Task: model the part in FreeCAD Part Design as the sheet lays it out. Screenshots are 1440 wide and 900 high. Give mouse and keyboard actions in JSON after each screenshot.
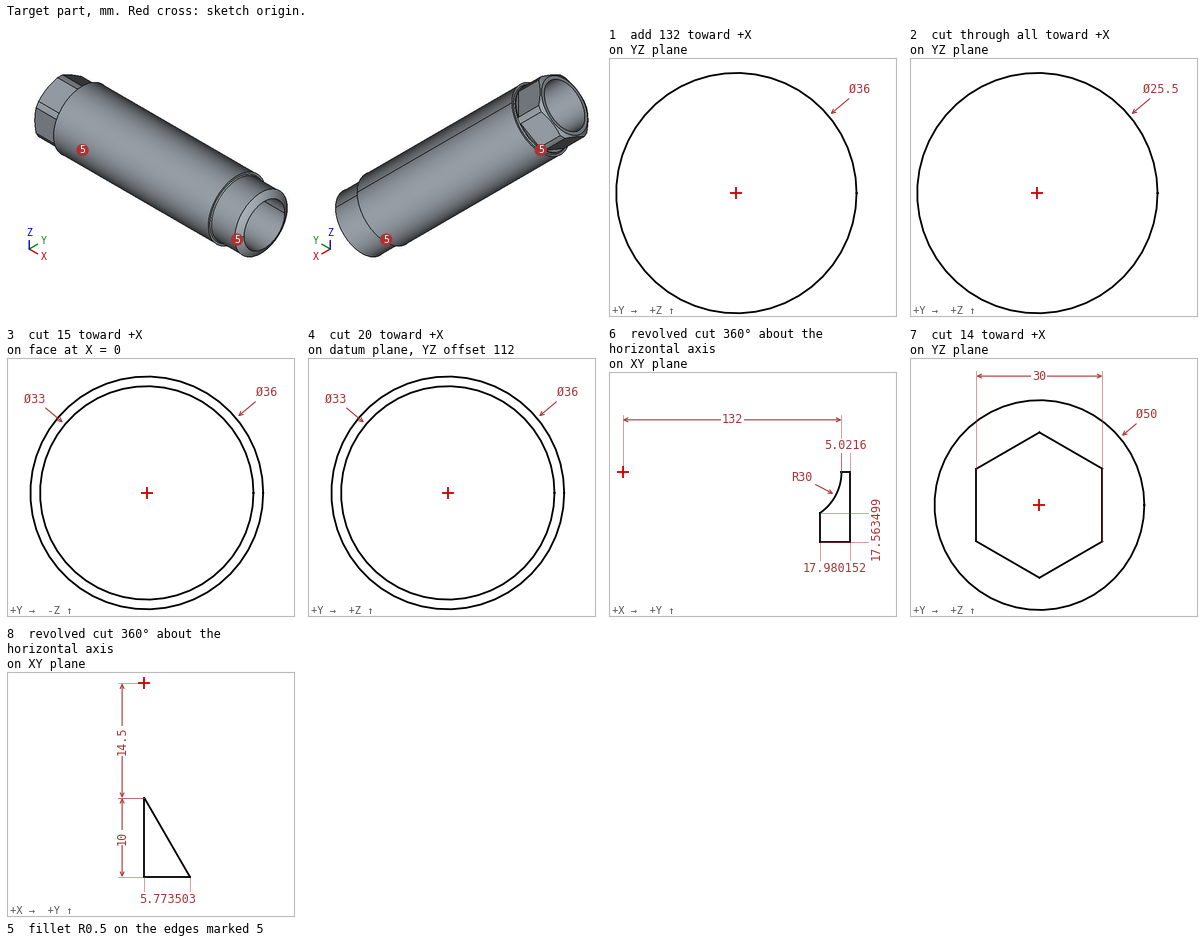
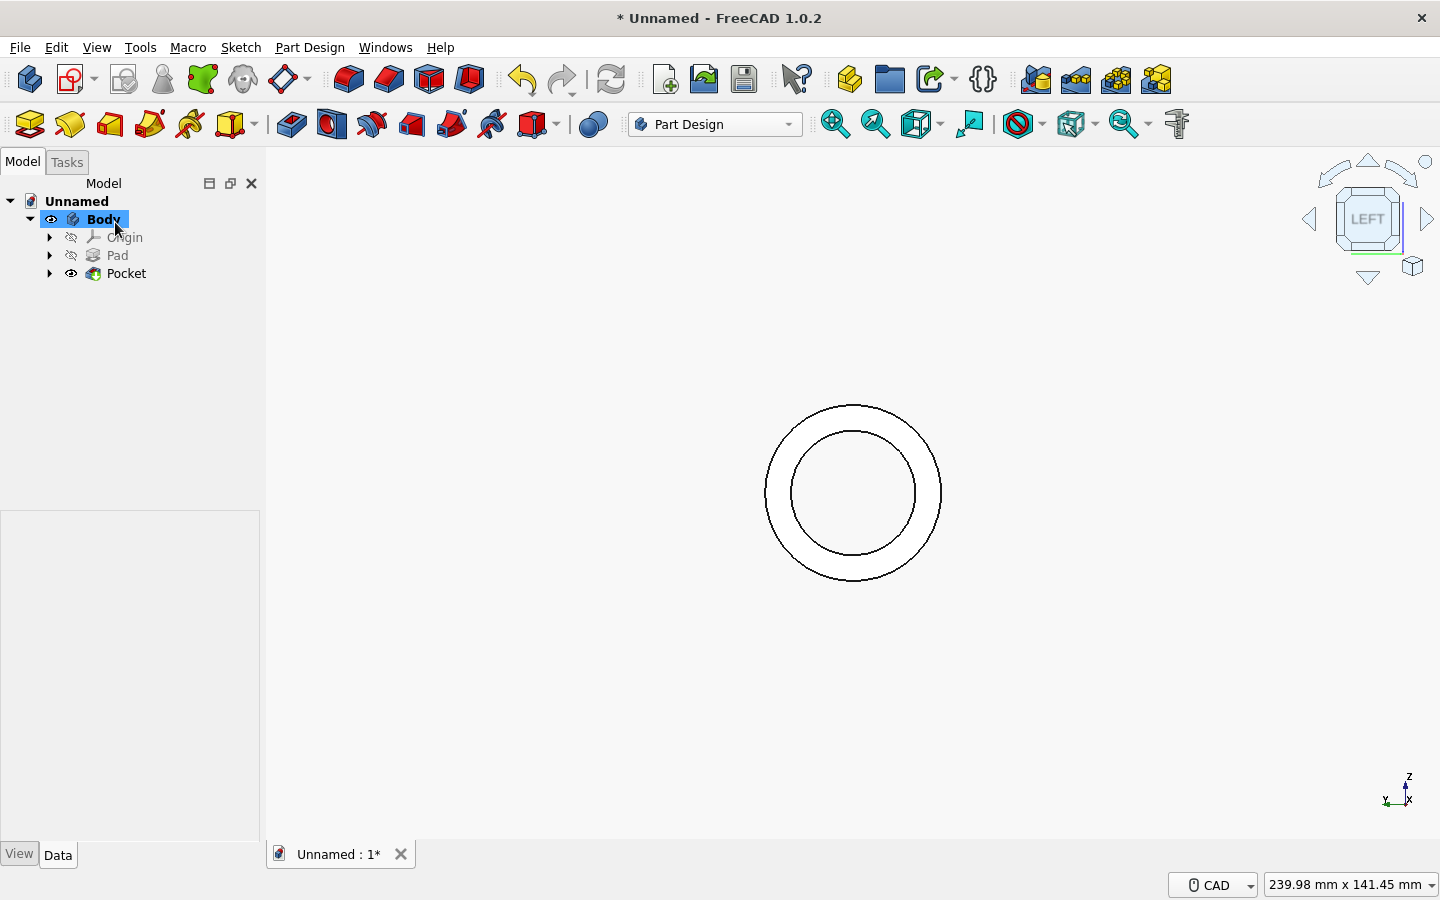
{"action": "key", "text": "v f"}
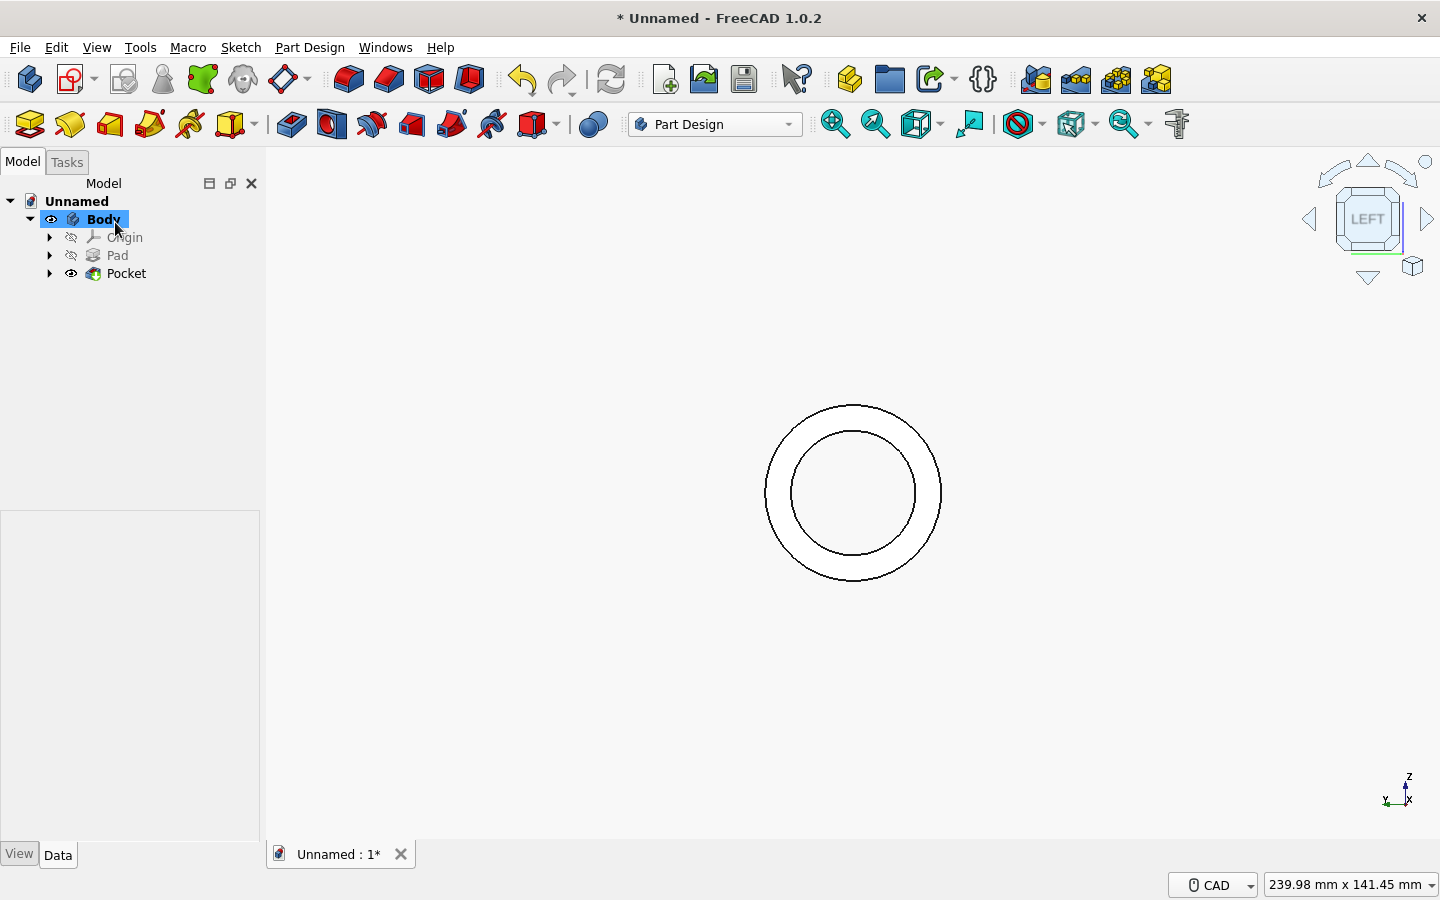
{"action": "left_click", "coordinate": [778, 492]}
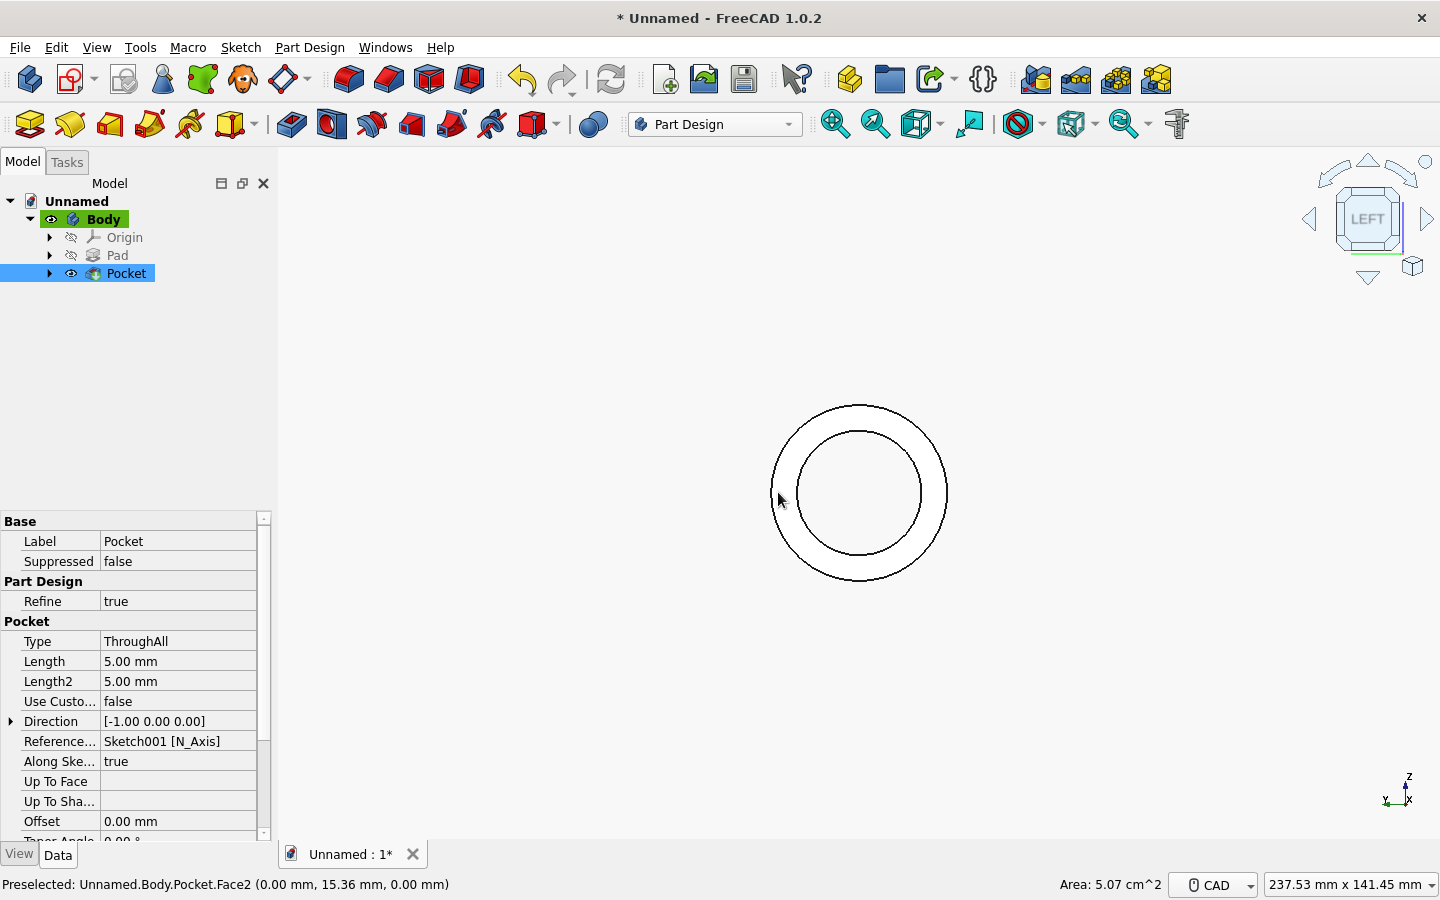
{"action": "left_click", "coordinate": [70, 80]}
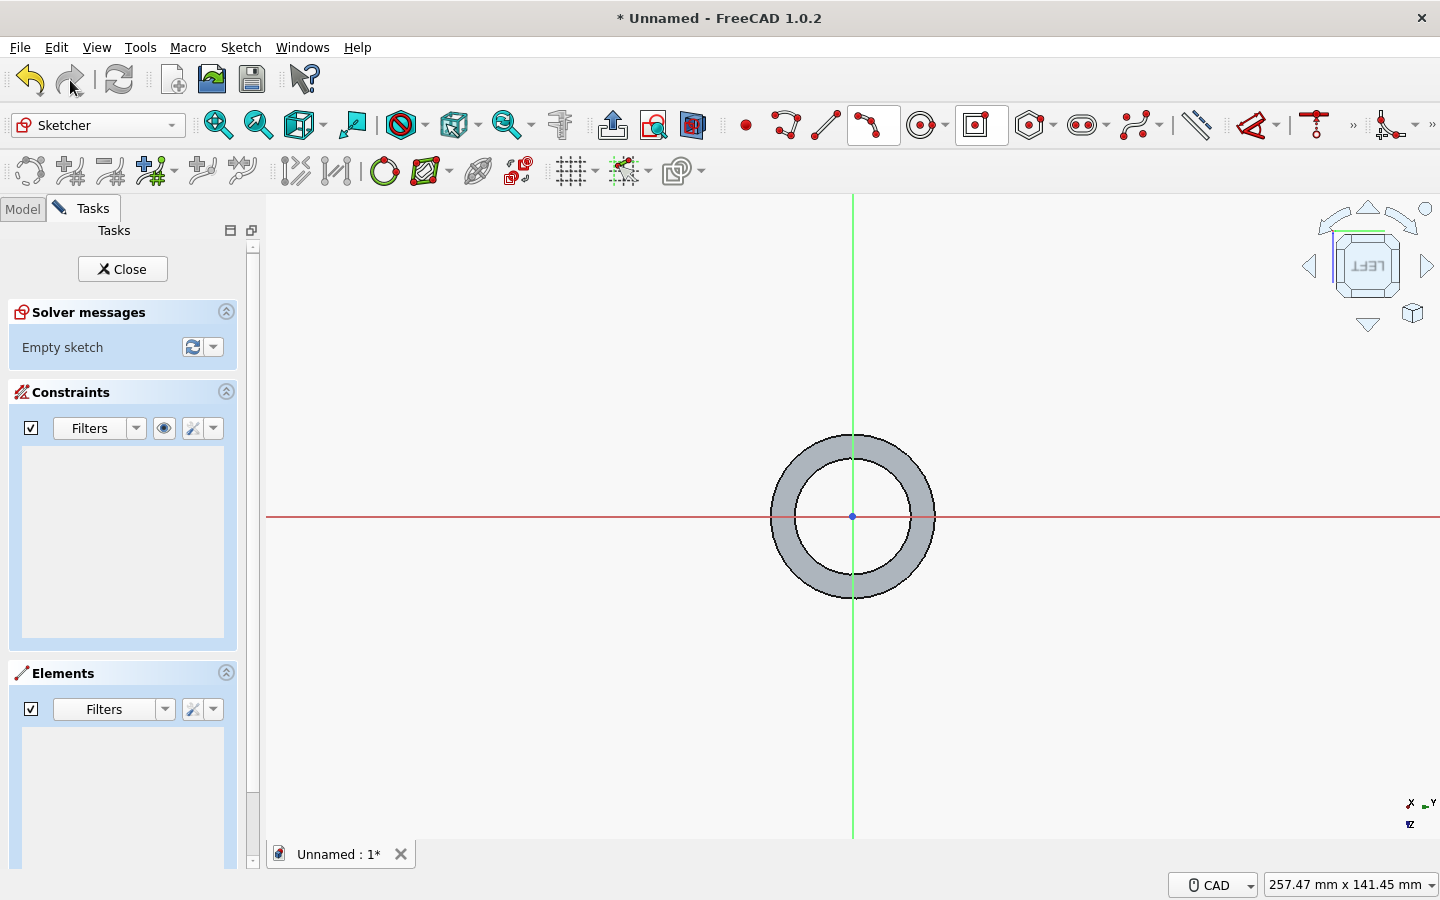
{"action": "scroll", "coordinate": [893, 516], "scroll_direction": "up", "scroll_amount": 5}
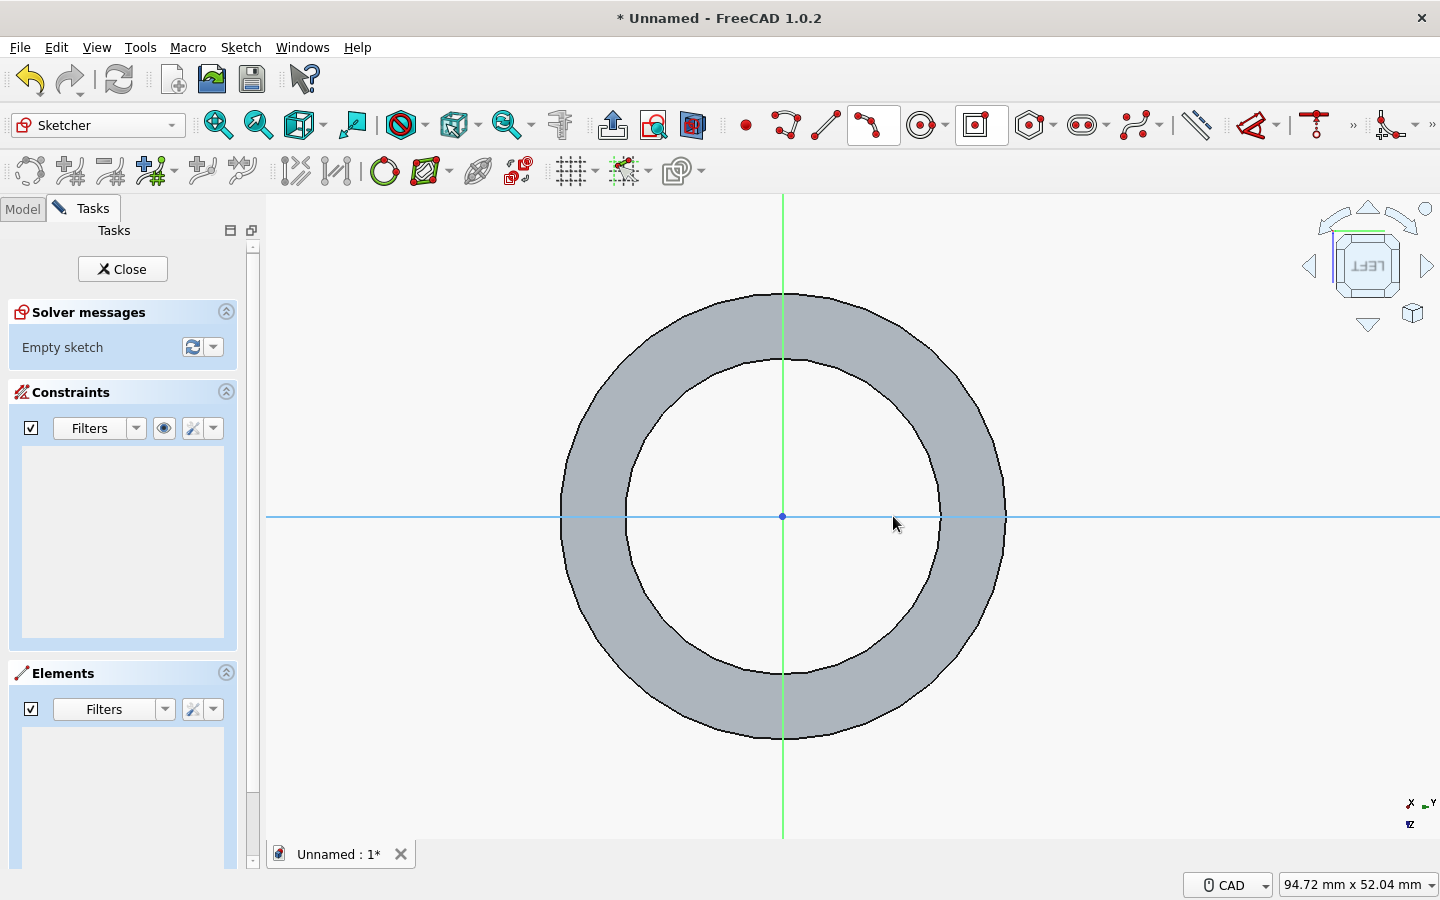
{"action": "key", "text": "g c"}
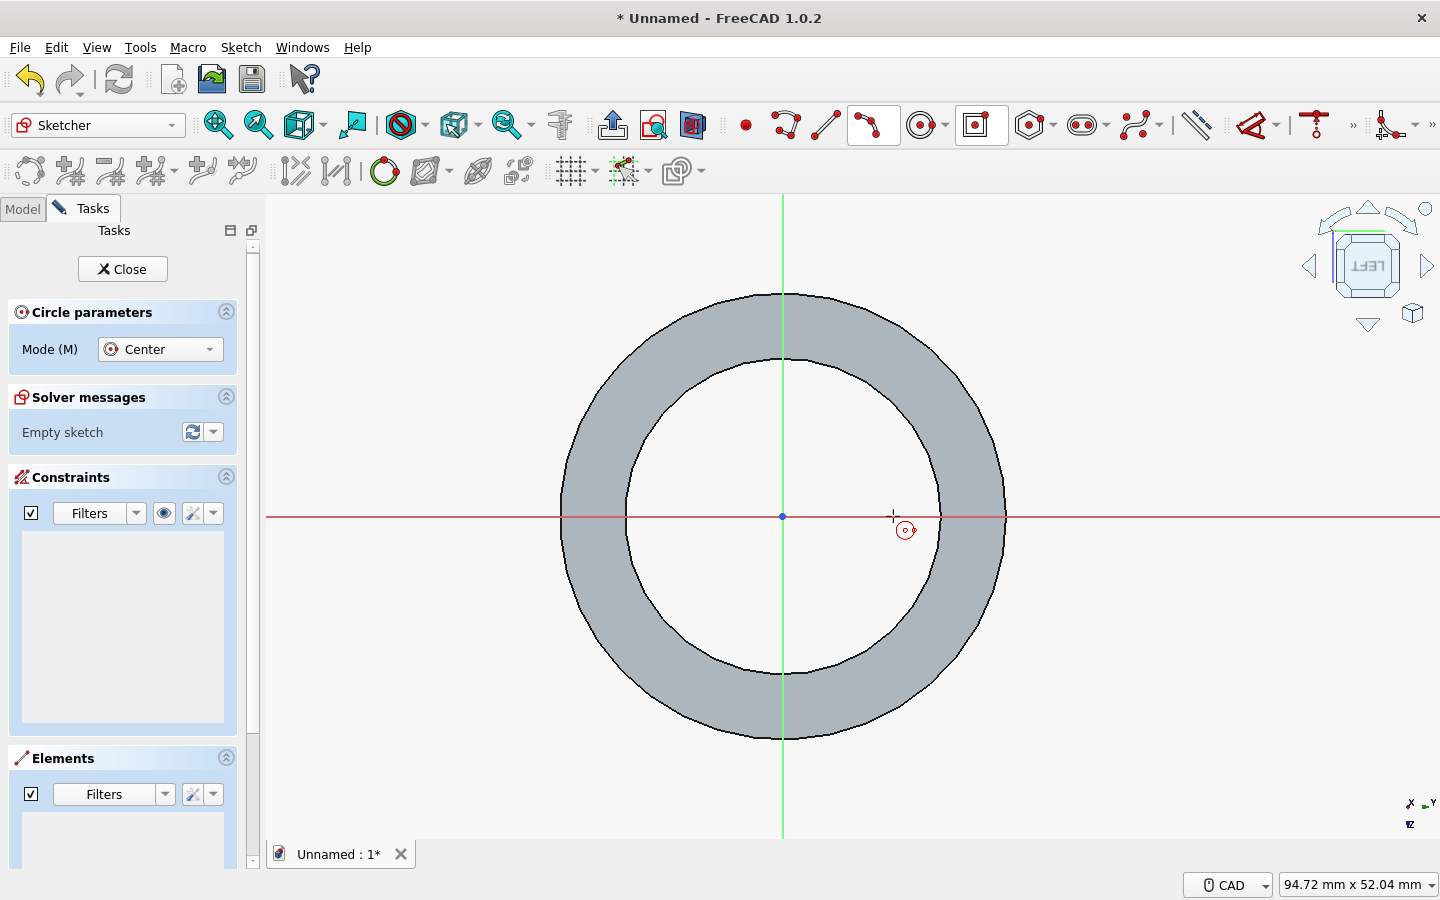
{"action": "left_click", "coordinate": [783, 516]}
{"action": "mouse_move", "coordinate": [941, 359]}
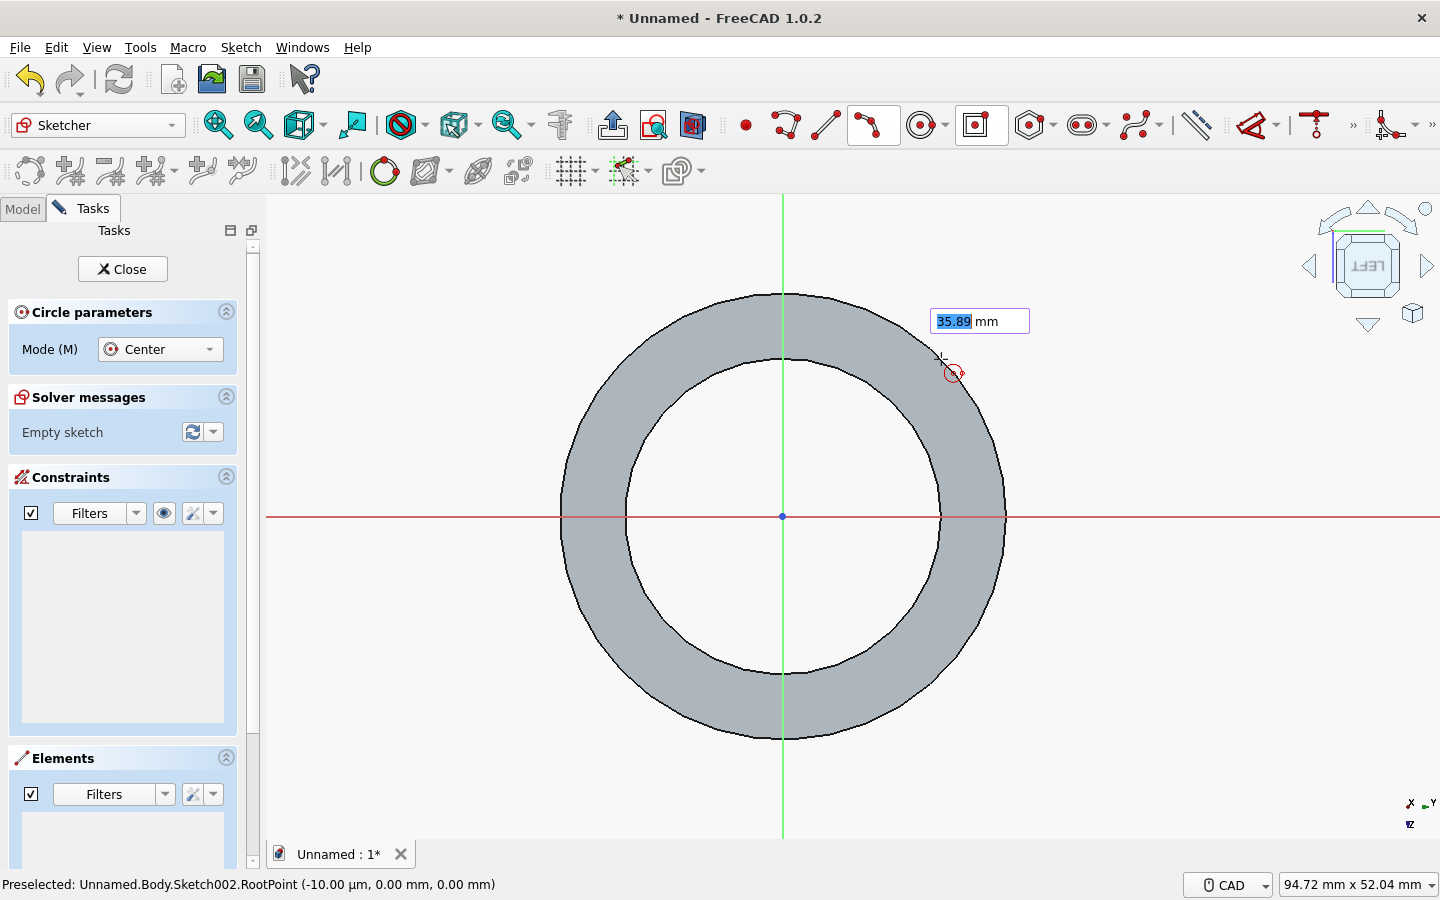
{"action": "type", "text": "36"}
{"action": "key", "text": "Return"}